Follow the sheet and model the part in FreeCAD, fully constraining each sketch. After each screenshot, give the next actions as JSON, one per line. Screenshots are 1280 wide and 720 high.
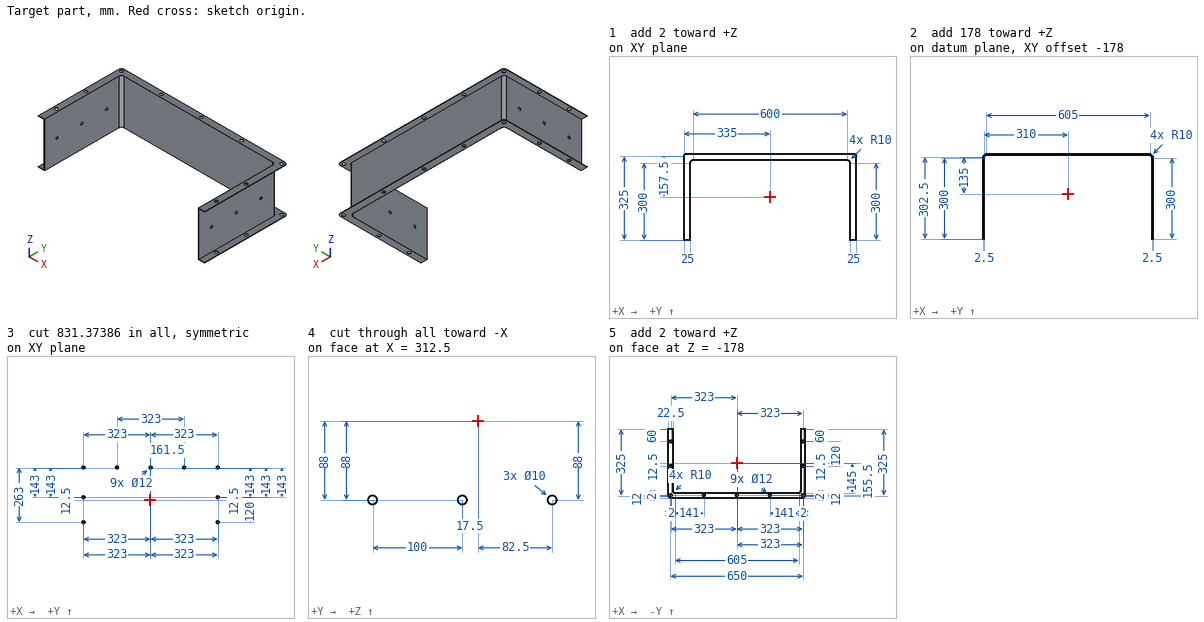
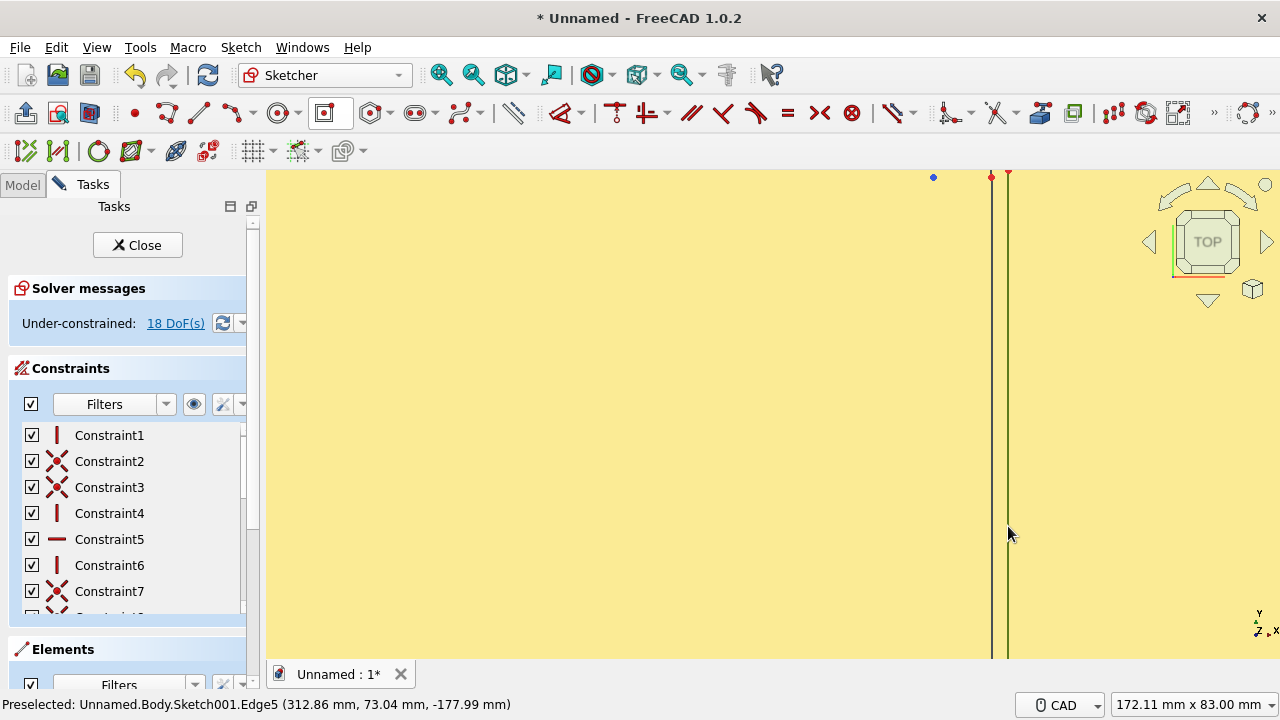
{"action": "scroll", "coordinate": [1009, 294], "scroll_direction": "down", "scroll_amount": 9}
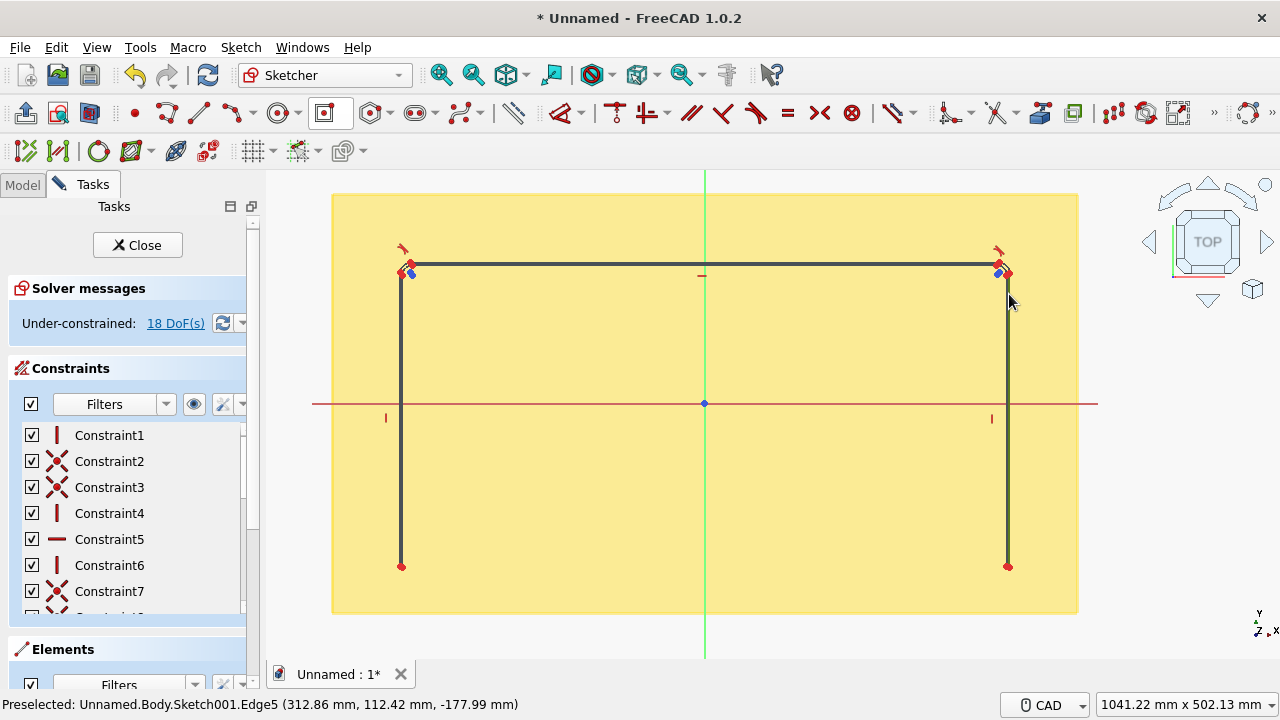
{"action": "scroll", "coordinate": [1009, 269], "scroll_direction": "up", "scroll_amount": 7}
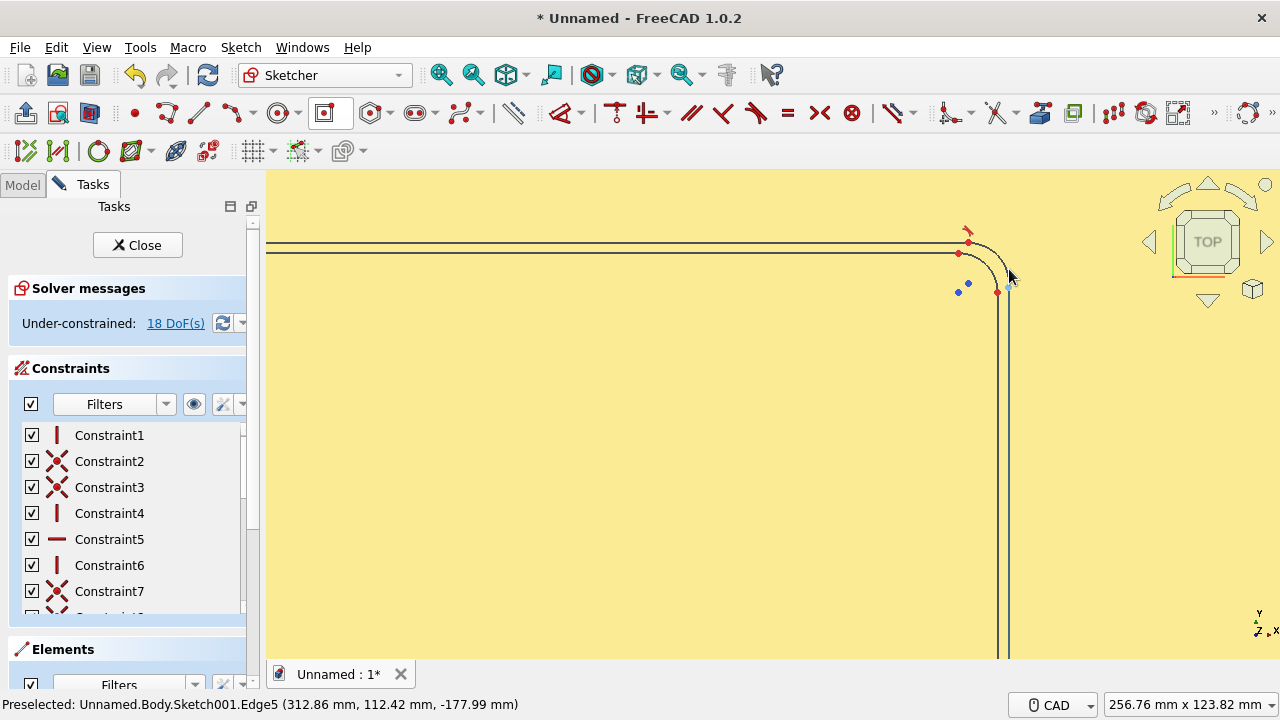
{"action": "left_click", "coordinate": [1006, 268]}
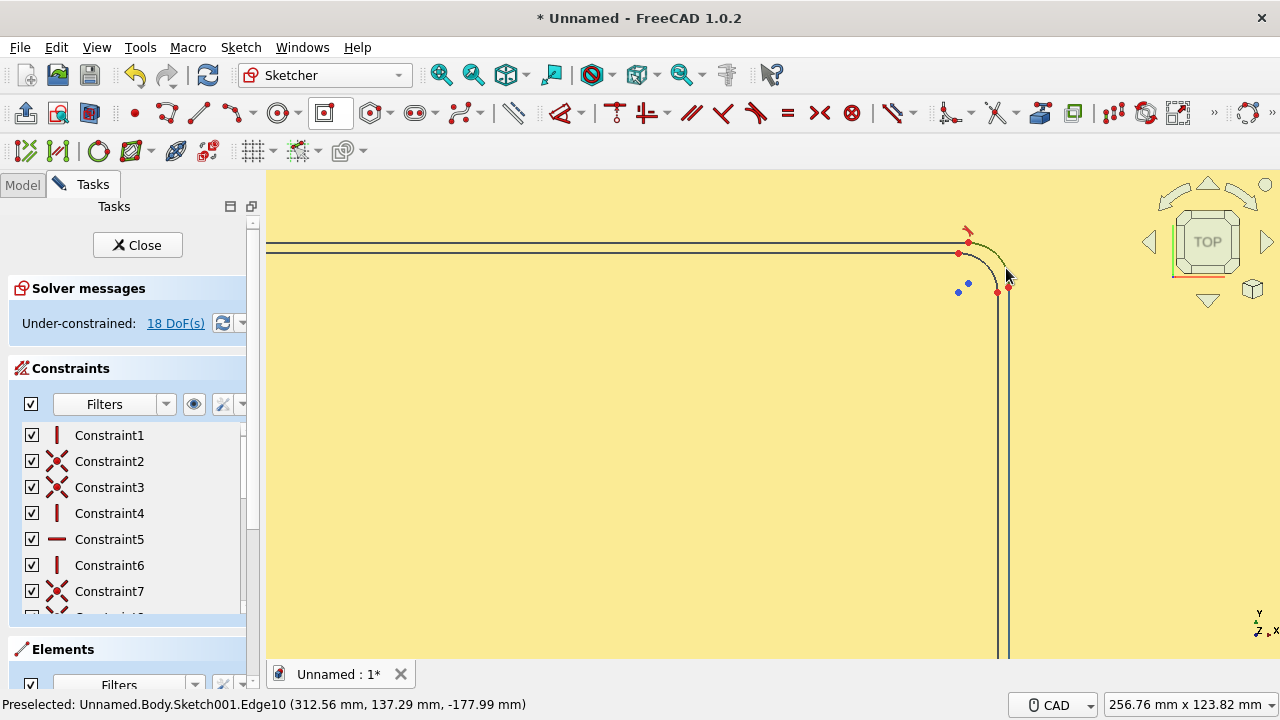
{"action": "left_click", "coordinate": [756, 114]}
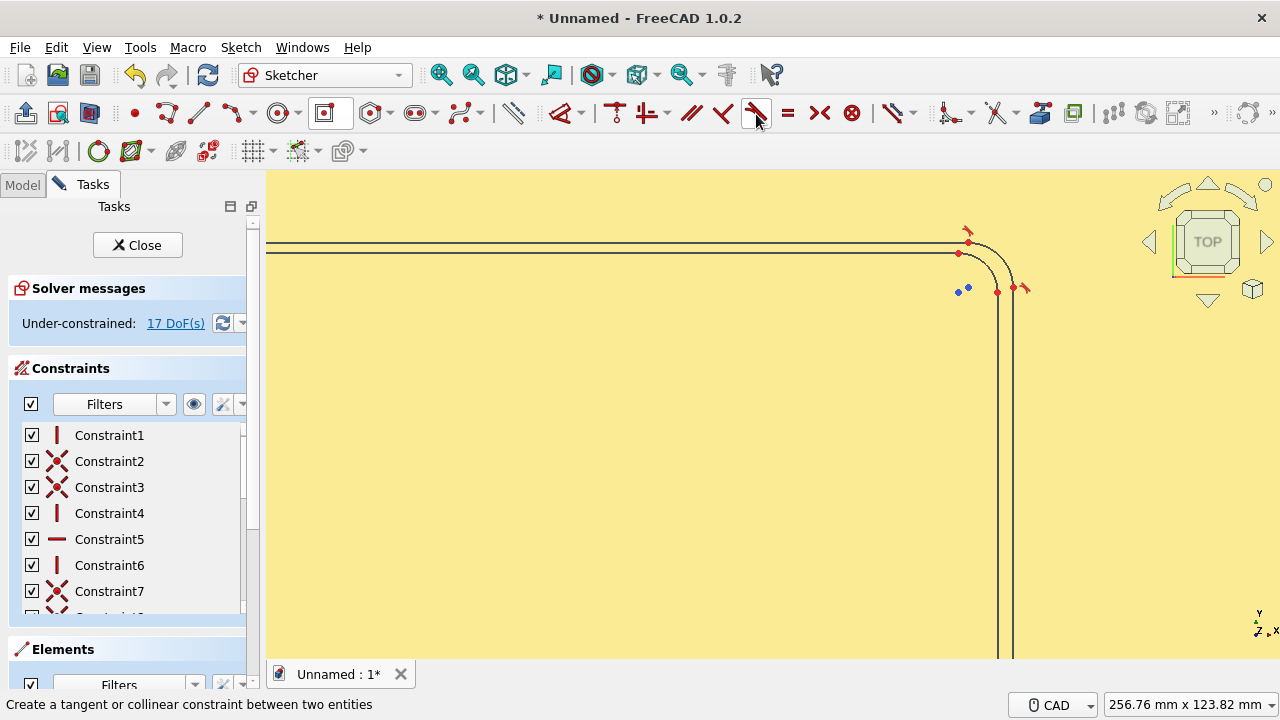
{"action": "left_click", "coordinate": [998, 530]}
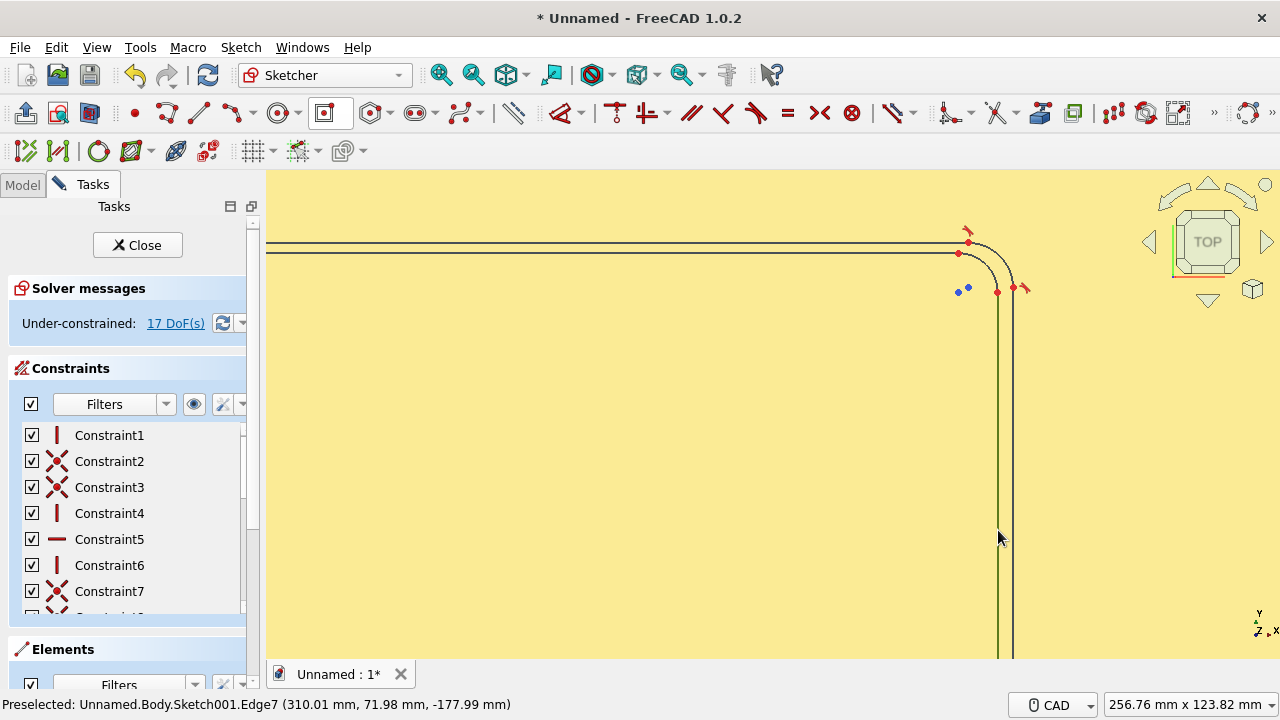
{"action": "left_click", "coordinate": [993, 275]}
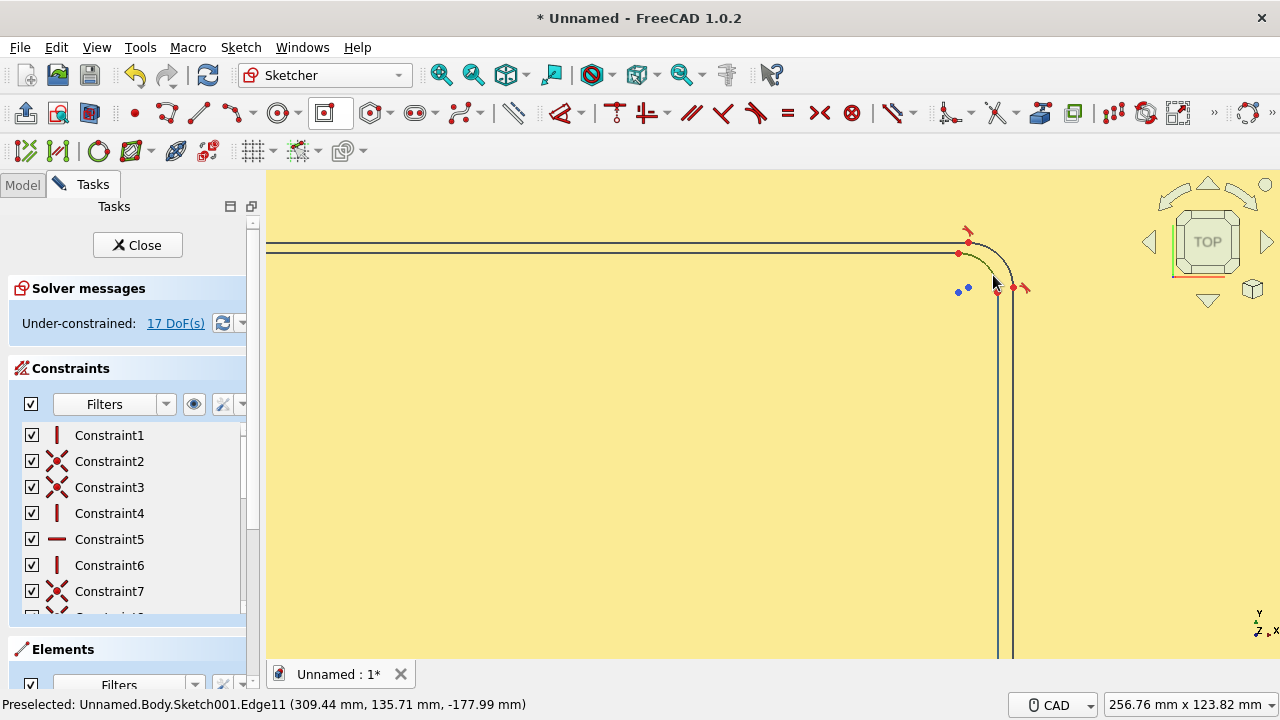
{"action": "left_click", "coordinate": [756, 114]}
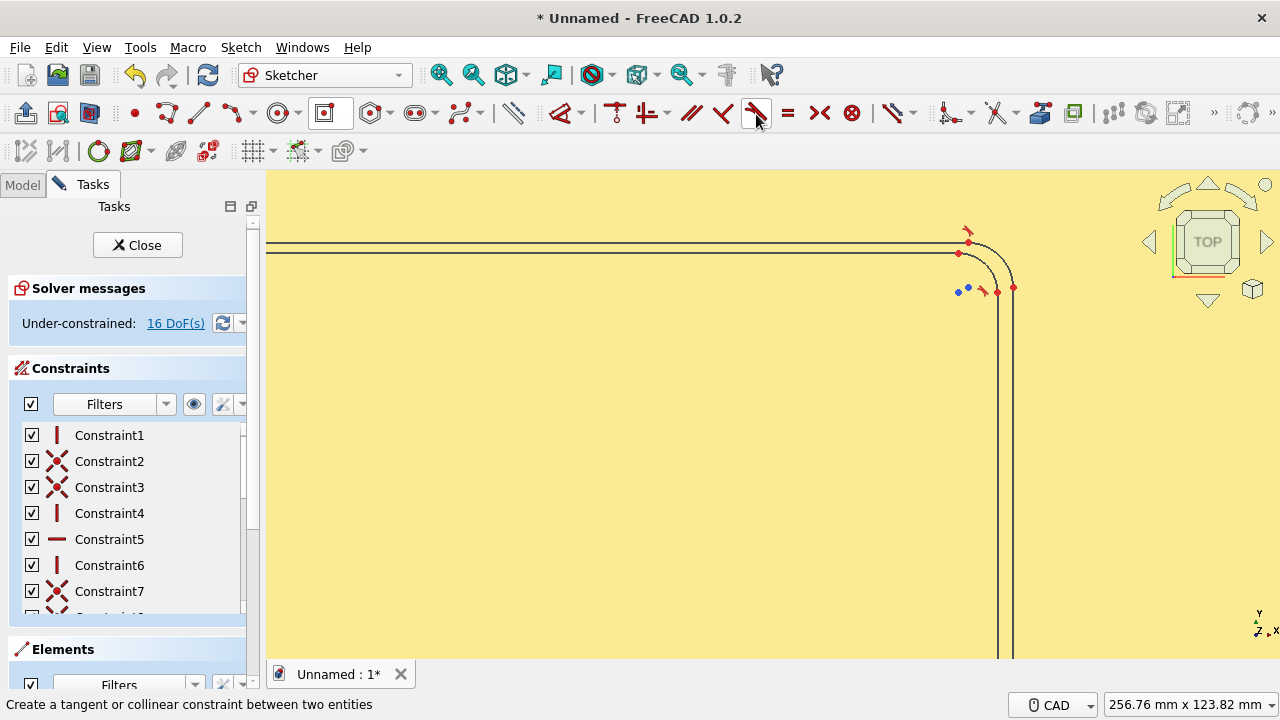
{"action": "scroll", "coordinate": [484, 253], "scroll_direction": "up", "scroll_amount": 2}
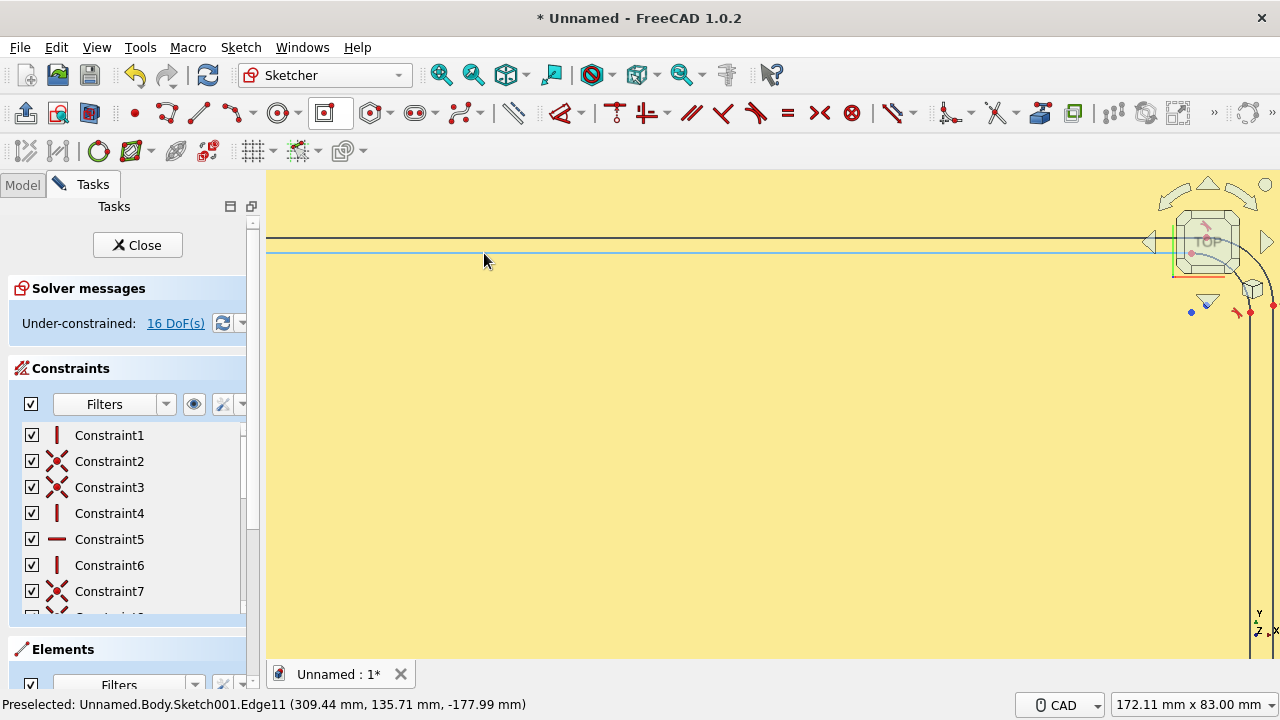
{"action": "left_click", "coordinate": [484, 253]}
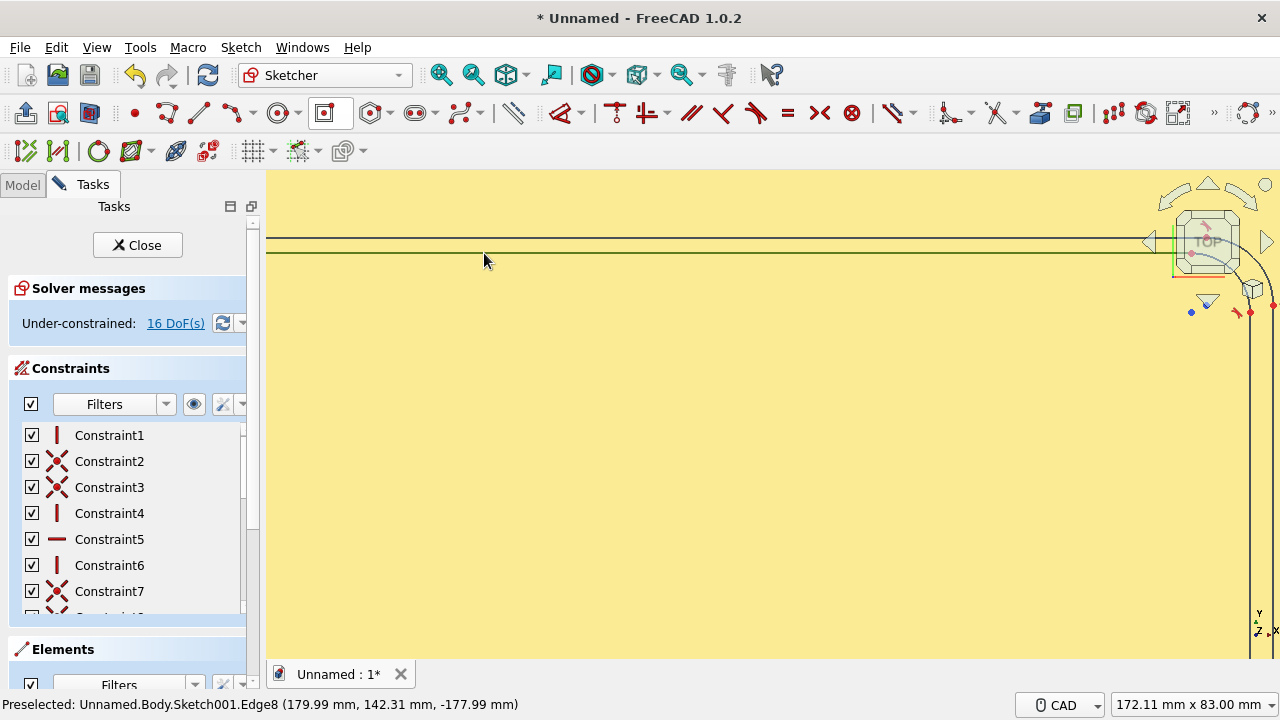
{"action": "scroll", "coordinate": [958, 267], "scroll_direction": "down", "scroll_amount": 9}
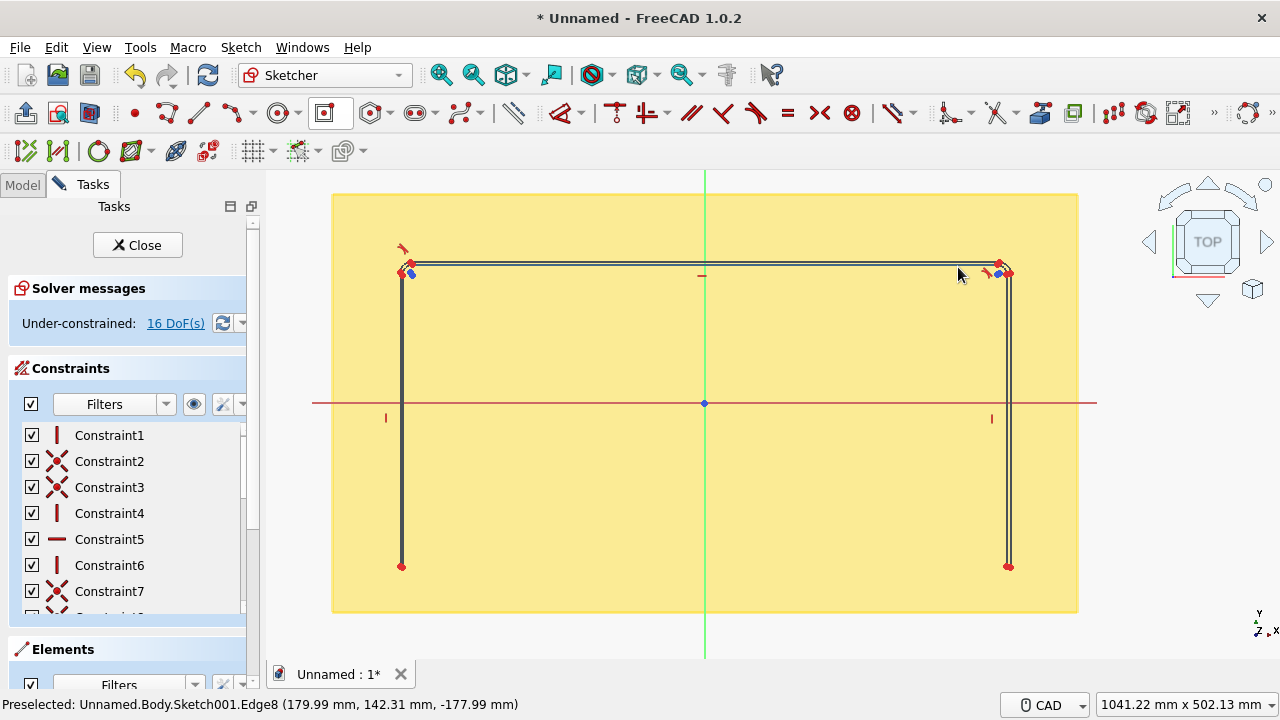
{"action": "scroll", "coordinate": [1006, 270], "scroll_direction": "up", "scroll_amount": 7}